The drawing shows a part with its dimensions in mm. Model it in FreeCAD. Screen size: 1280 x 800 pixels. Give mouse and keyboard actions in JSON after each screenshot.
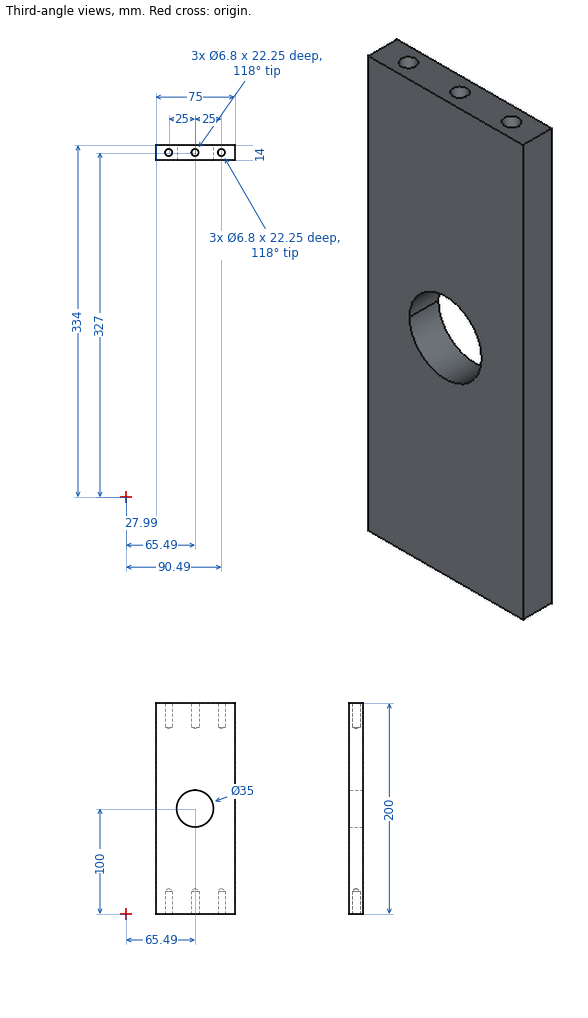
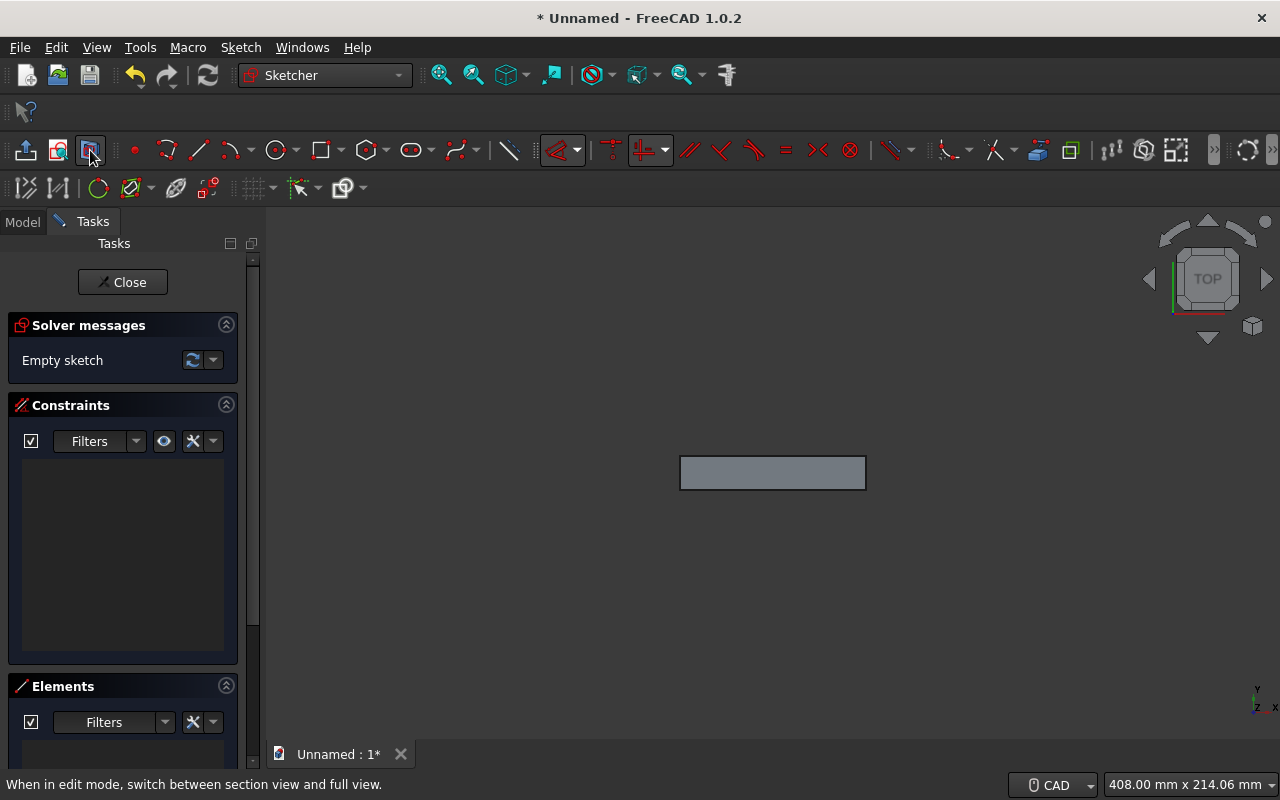
{"action": "scroll", "coordinate": [795, 473], "scroll_direction": "up", "scroll_amount": 7}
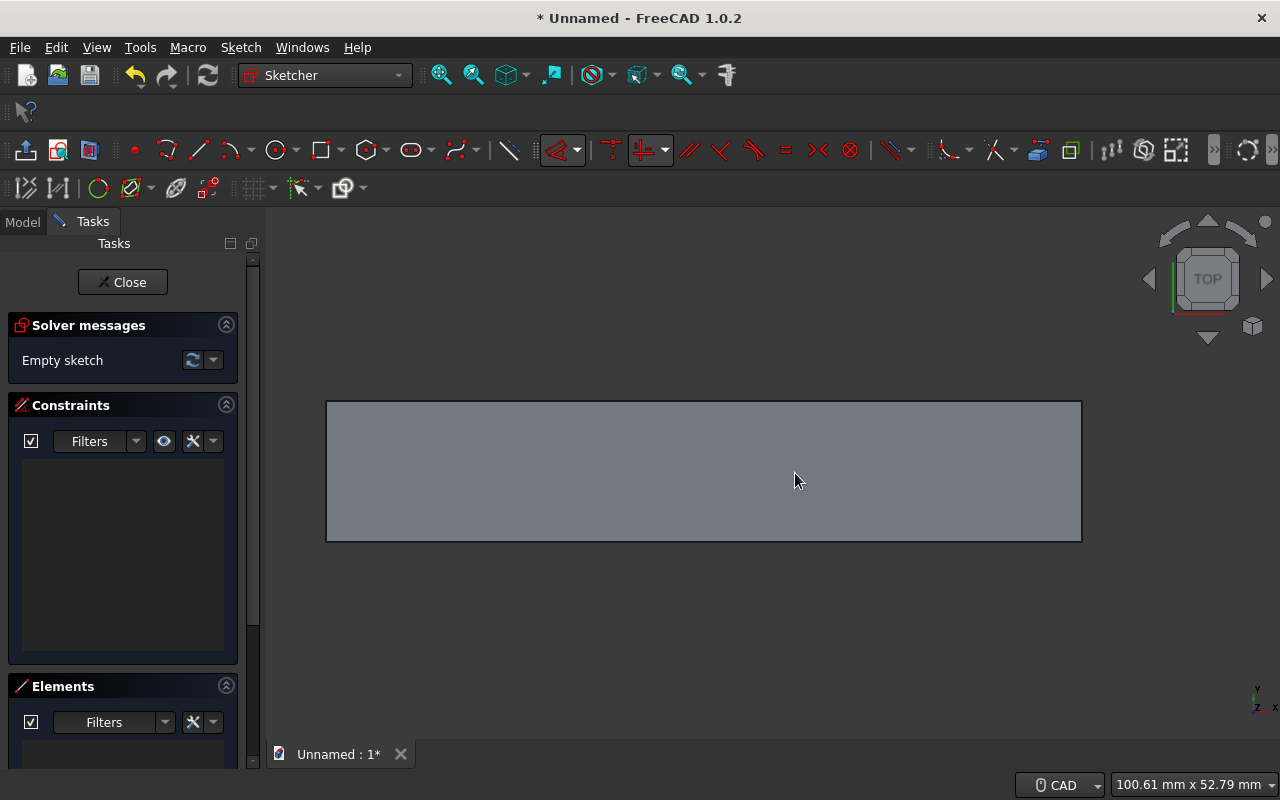
{"action": "left_click", "coordinate": [276, 150]}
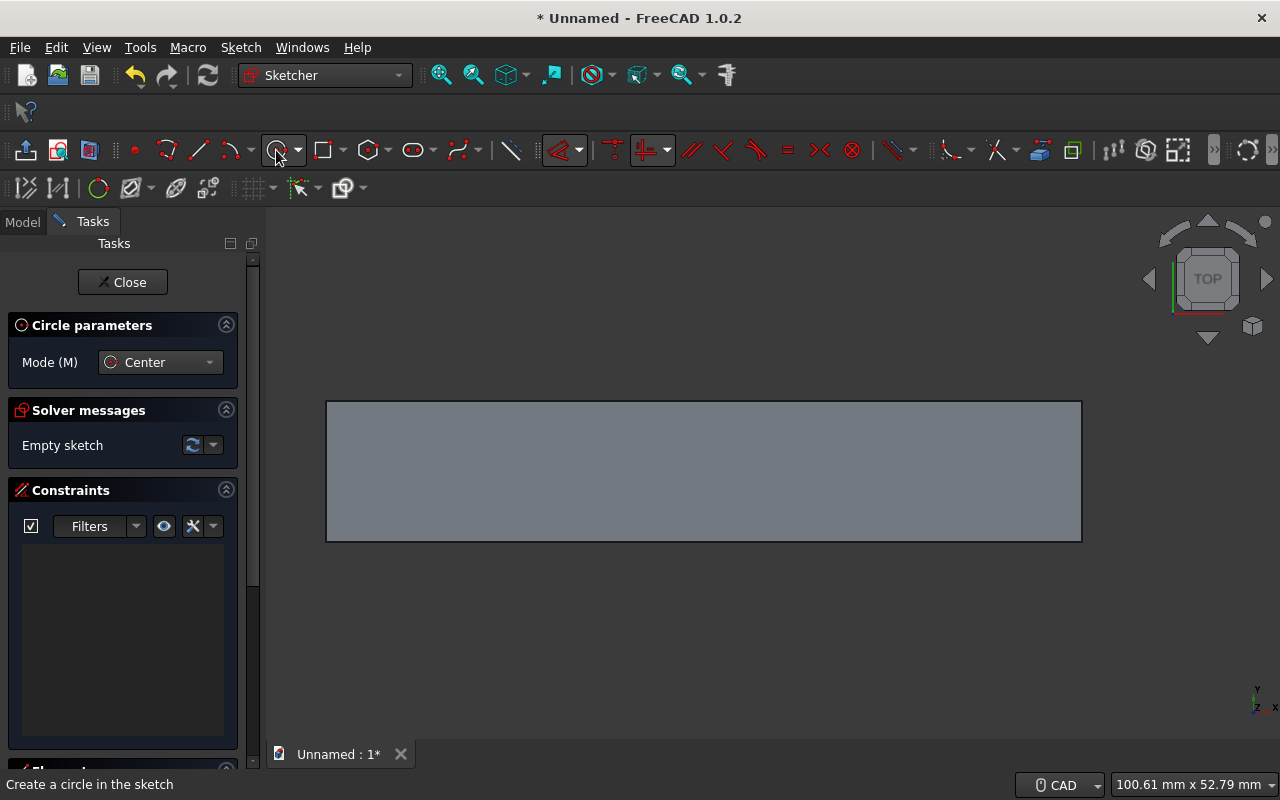
{"action": "left_click", "coordinate": [956, 471]}
{"action": "mouse_move", "coordinate": [980, 447]}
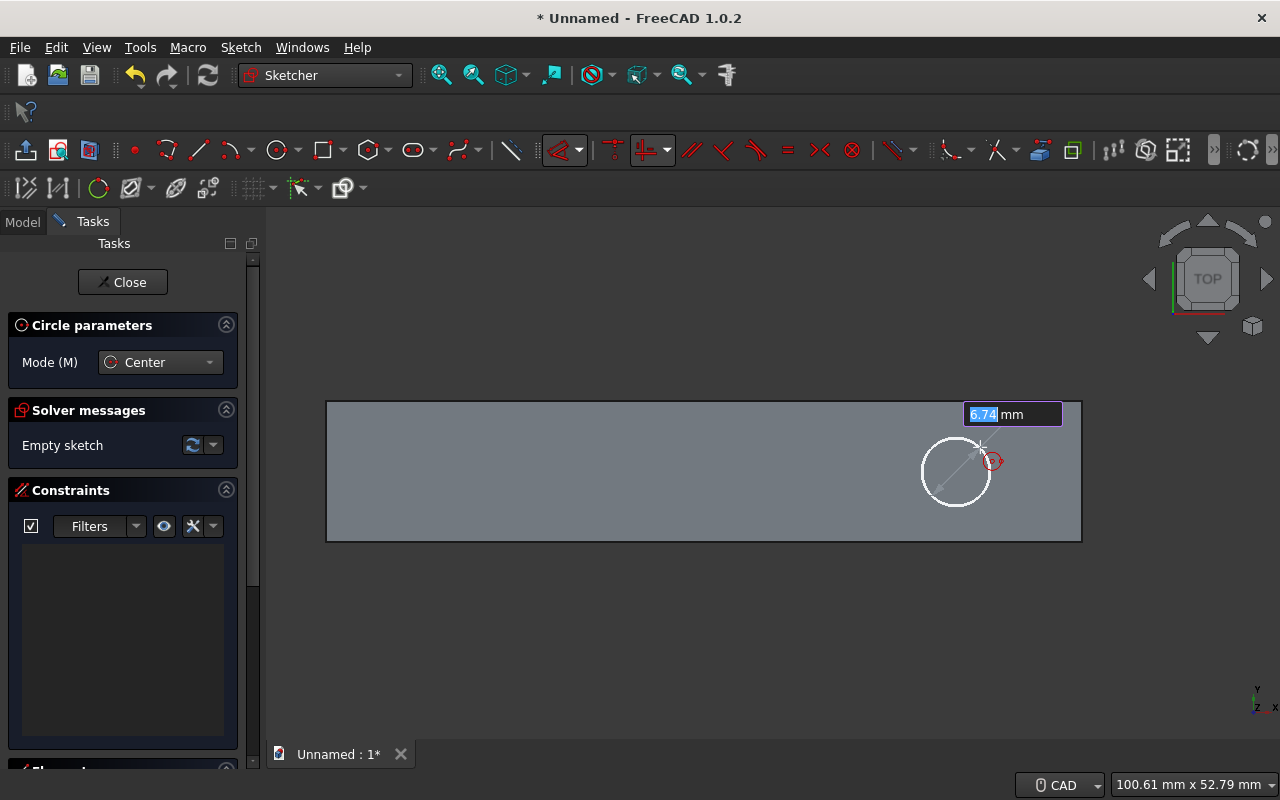
{"action": "type", "text": "6.8"}
{"action": "key", "text": "Return"}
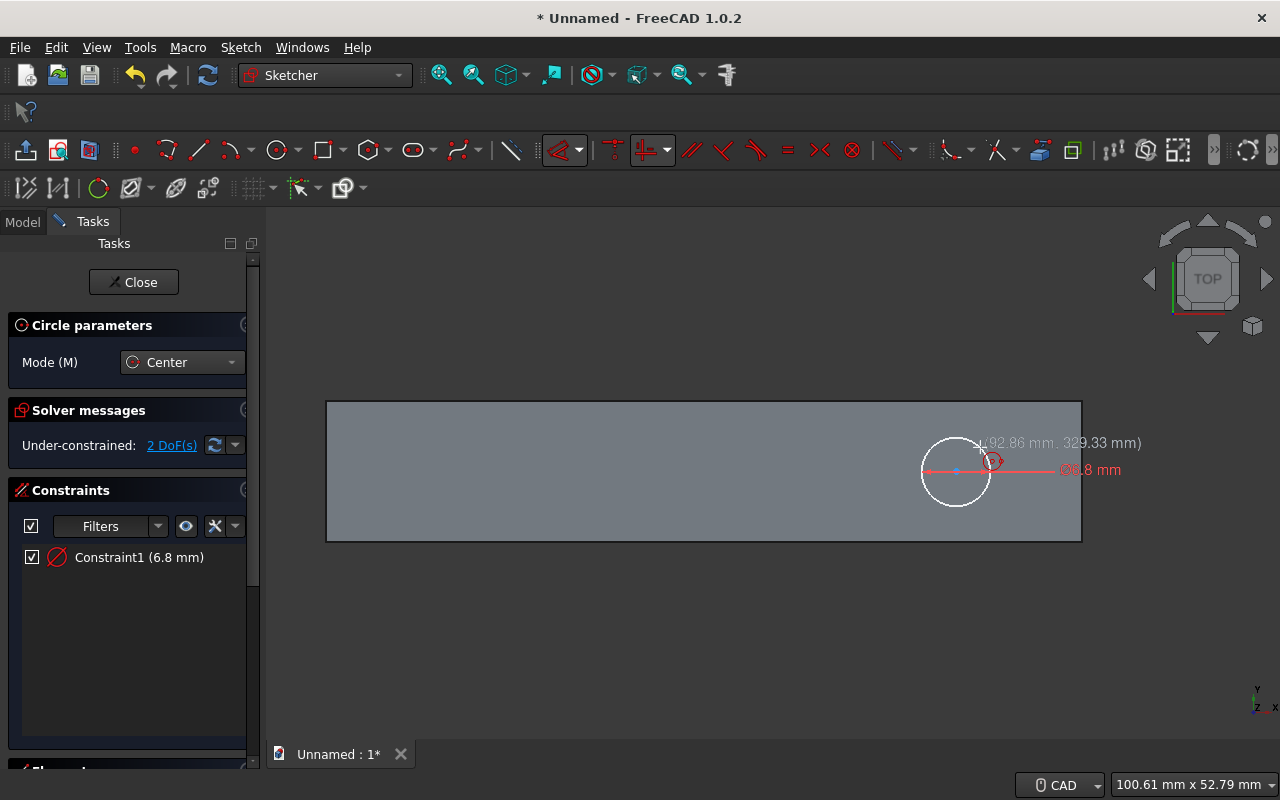
{"action": "left_click", "coordinate": [704, 471]}
{"action": "mouse_move", "coordinate": [728, 447]}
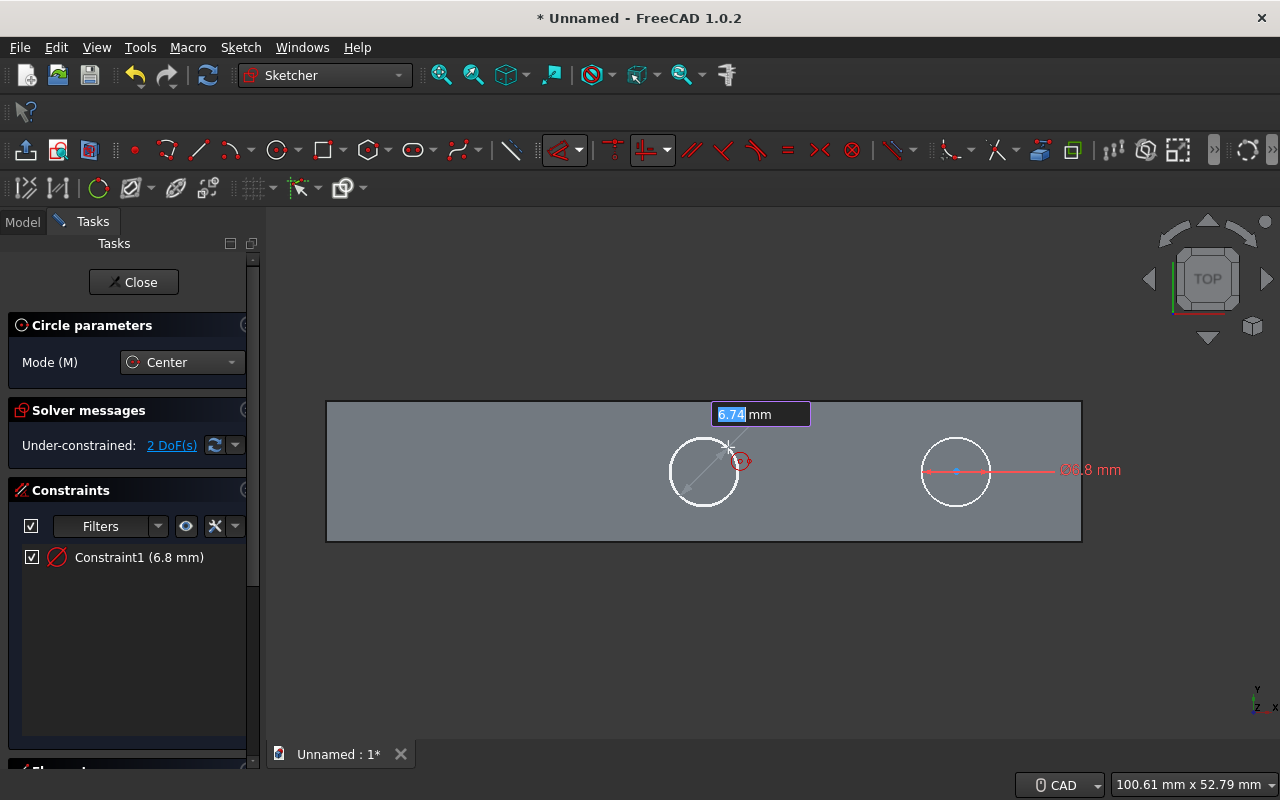
{"action": "type", "text": "6.8"}
{"action": "key", "text": "Return"}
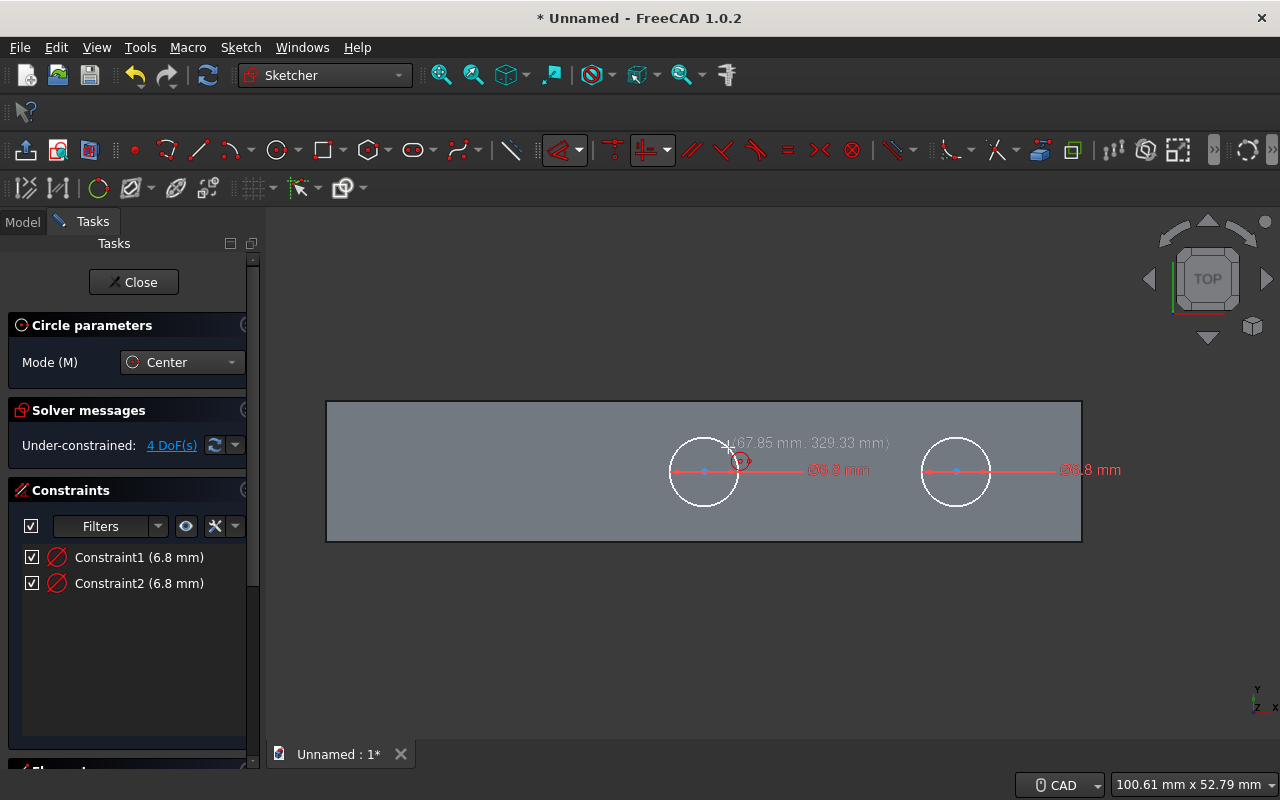
{"action": "left_click", "coordinate": [452, 471]}
{"action": "mouse_move", "coordinate": [476, 447]}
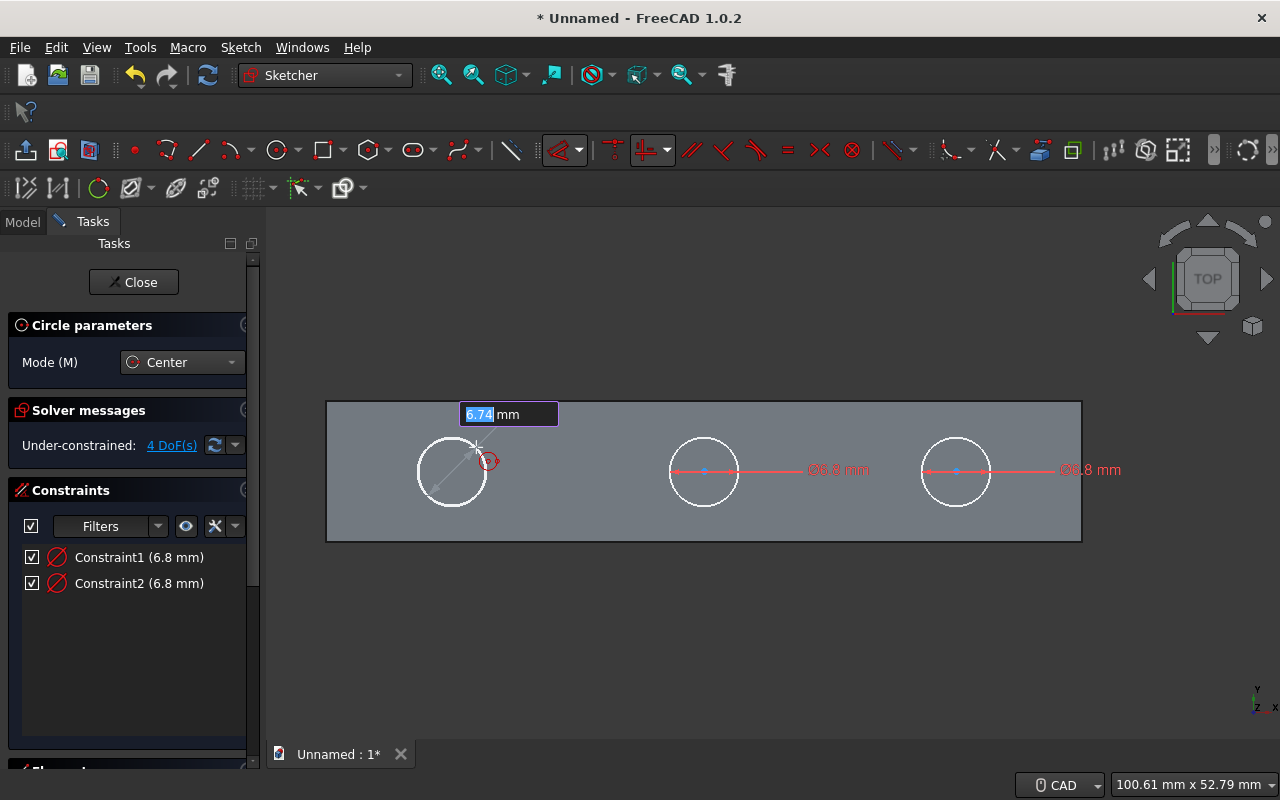
{"action": "type", "text": "6.8"}
{"action": "key", "text": "Return"}
{"action": "key", "text": "Escape"}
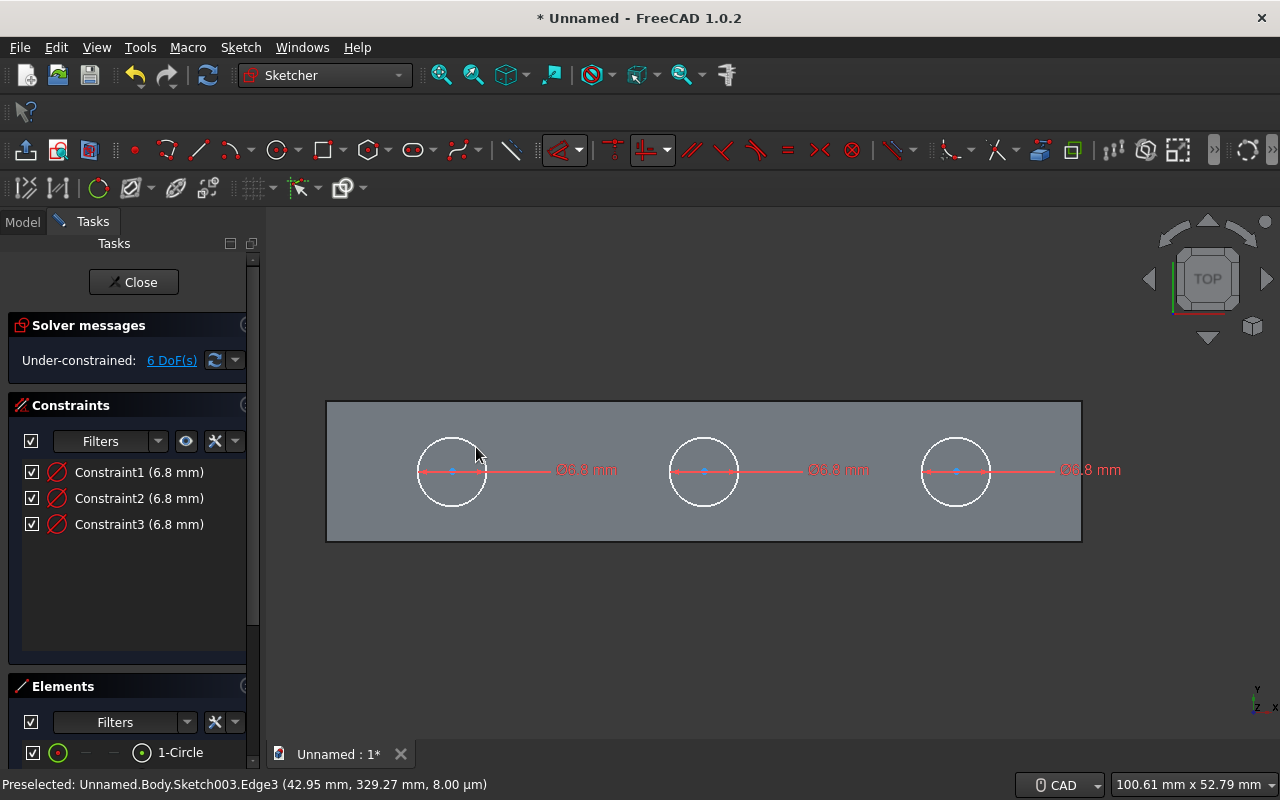
{"action": "left_click", "coordinate": [956, 472]}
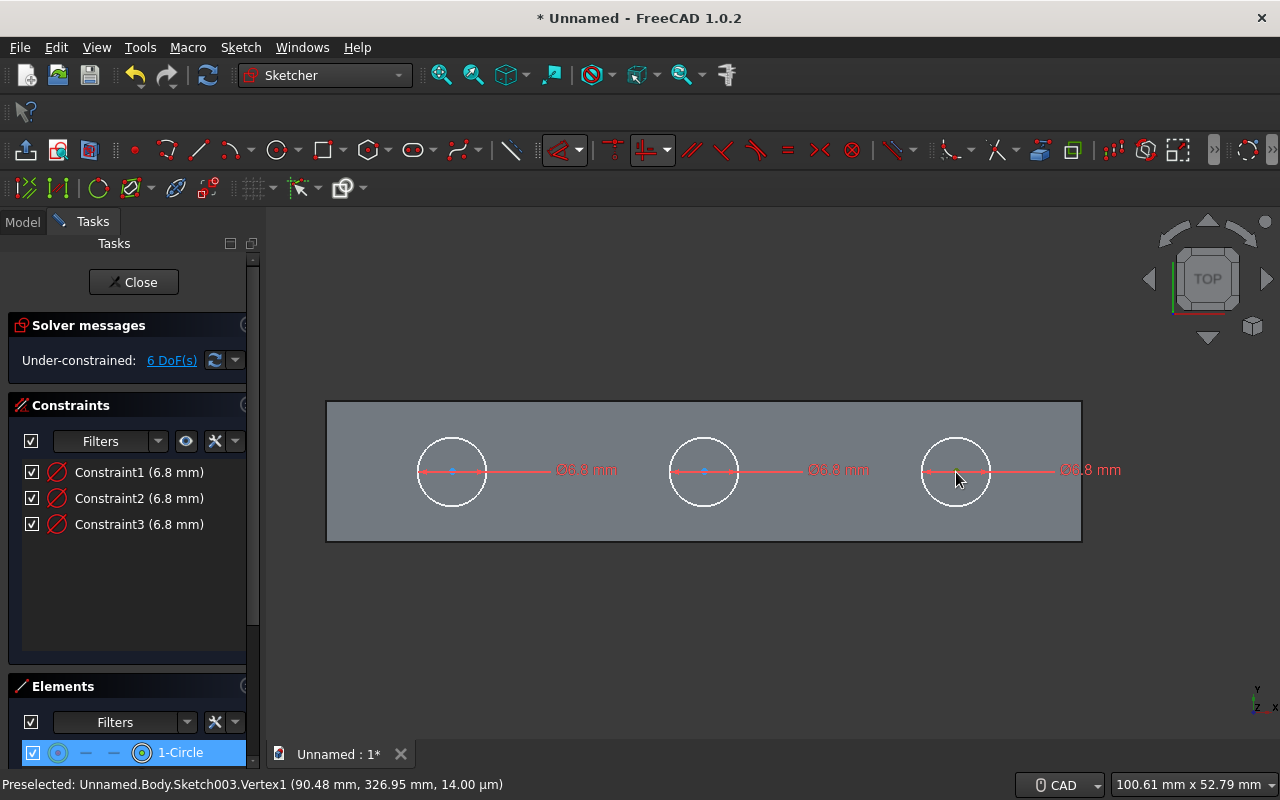
{"action": "left_click", "coordinate": [704, 472]}